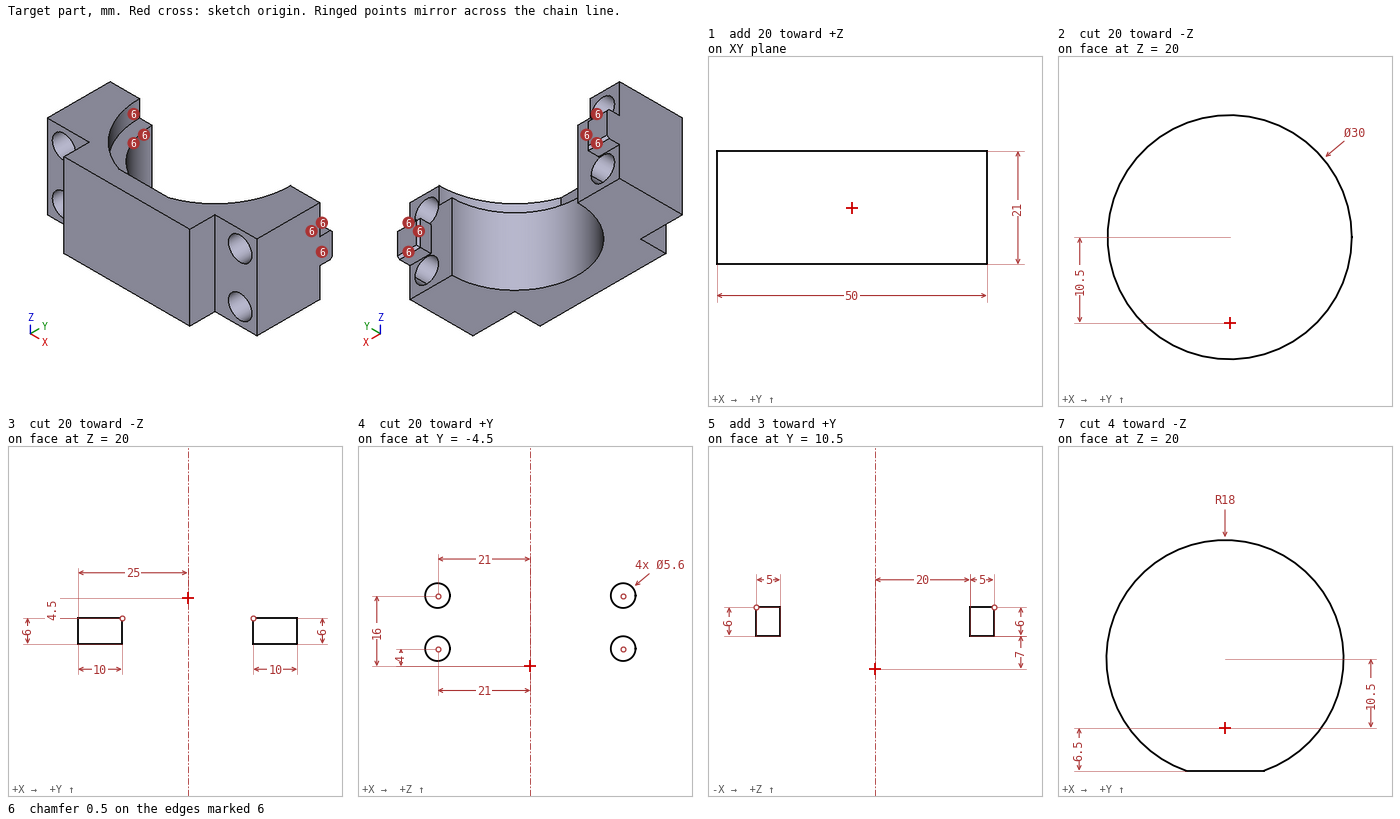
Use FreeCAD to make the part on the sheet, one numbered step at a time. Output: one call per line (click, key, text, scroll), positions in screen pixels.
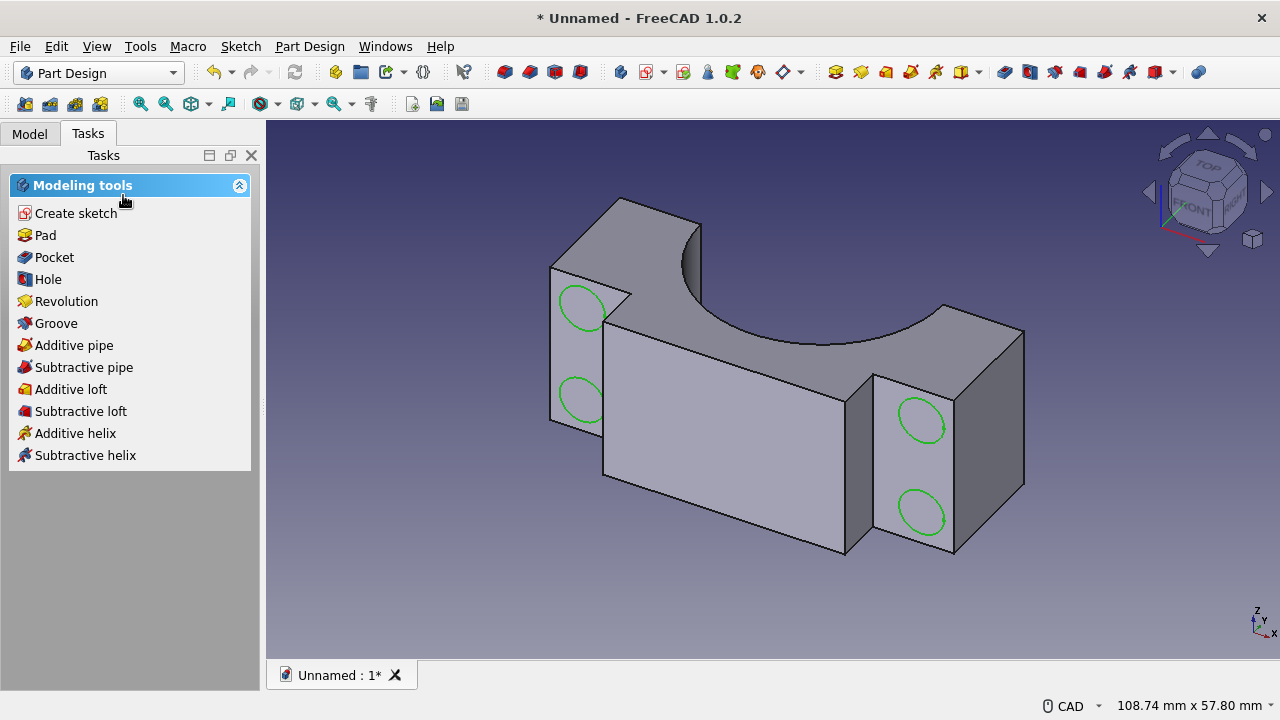
click(1005, 72)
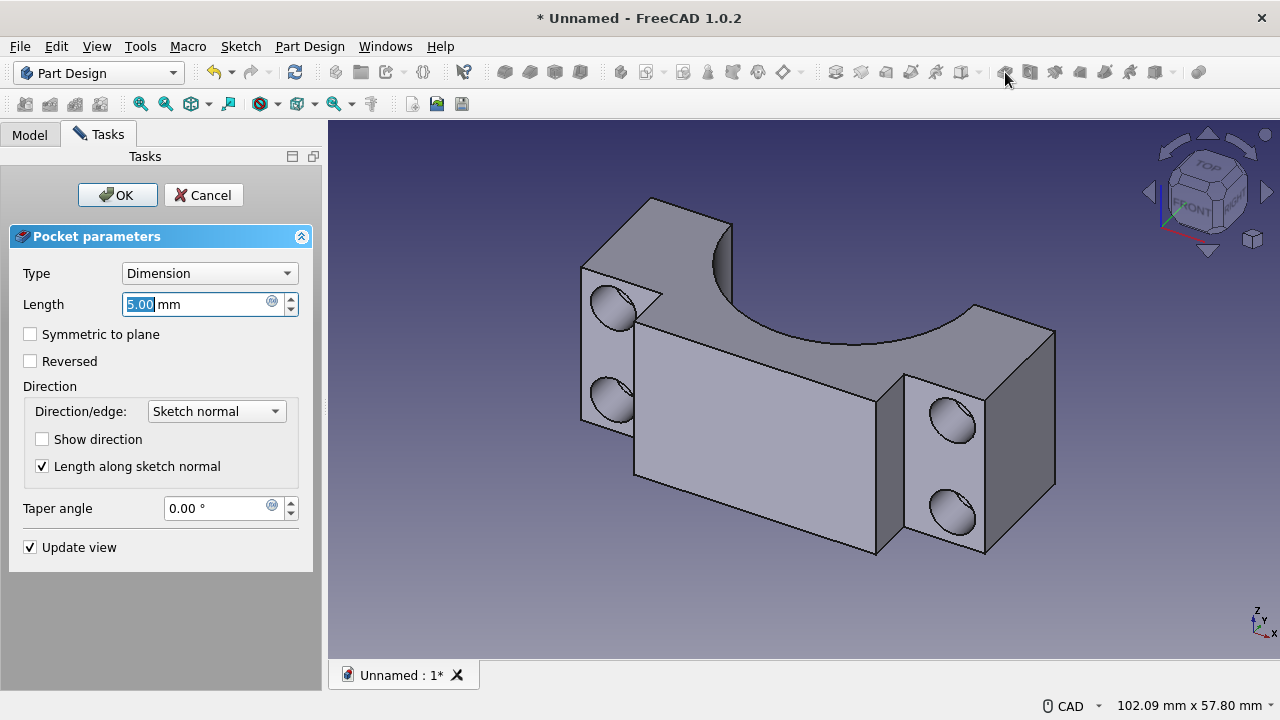
text(20)
key(Tab)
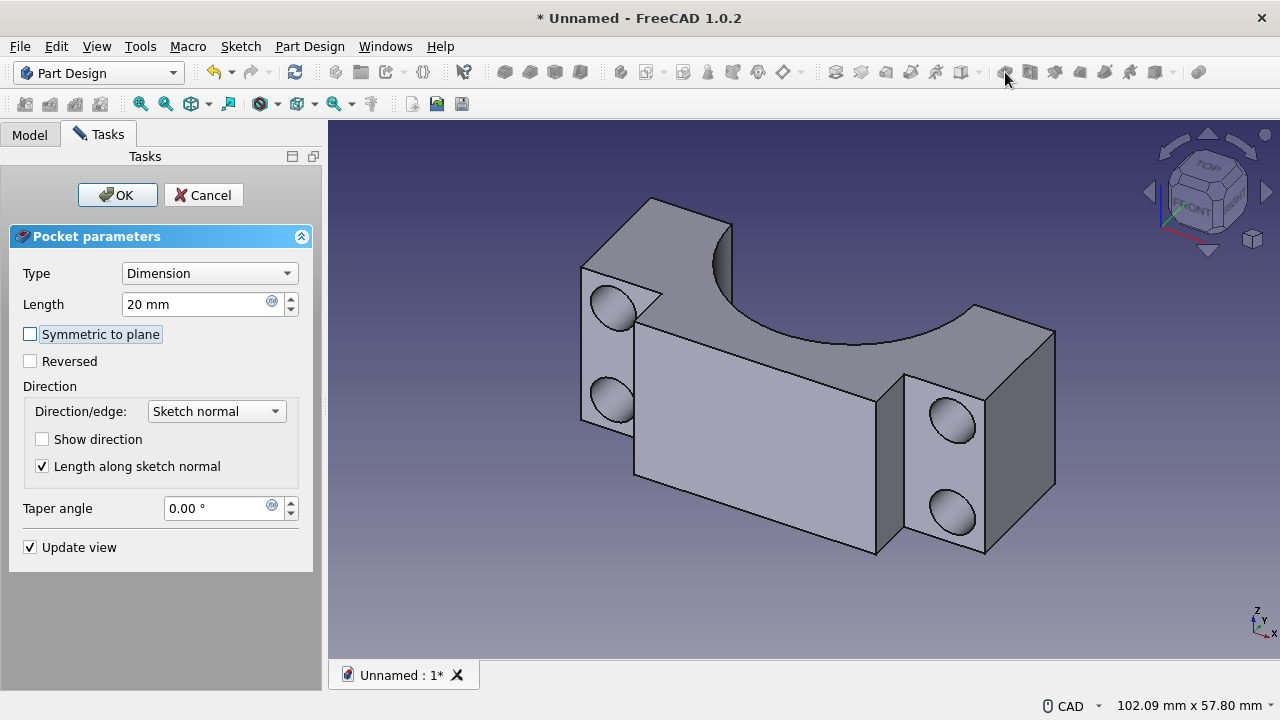
click(118, 195)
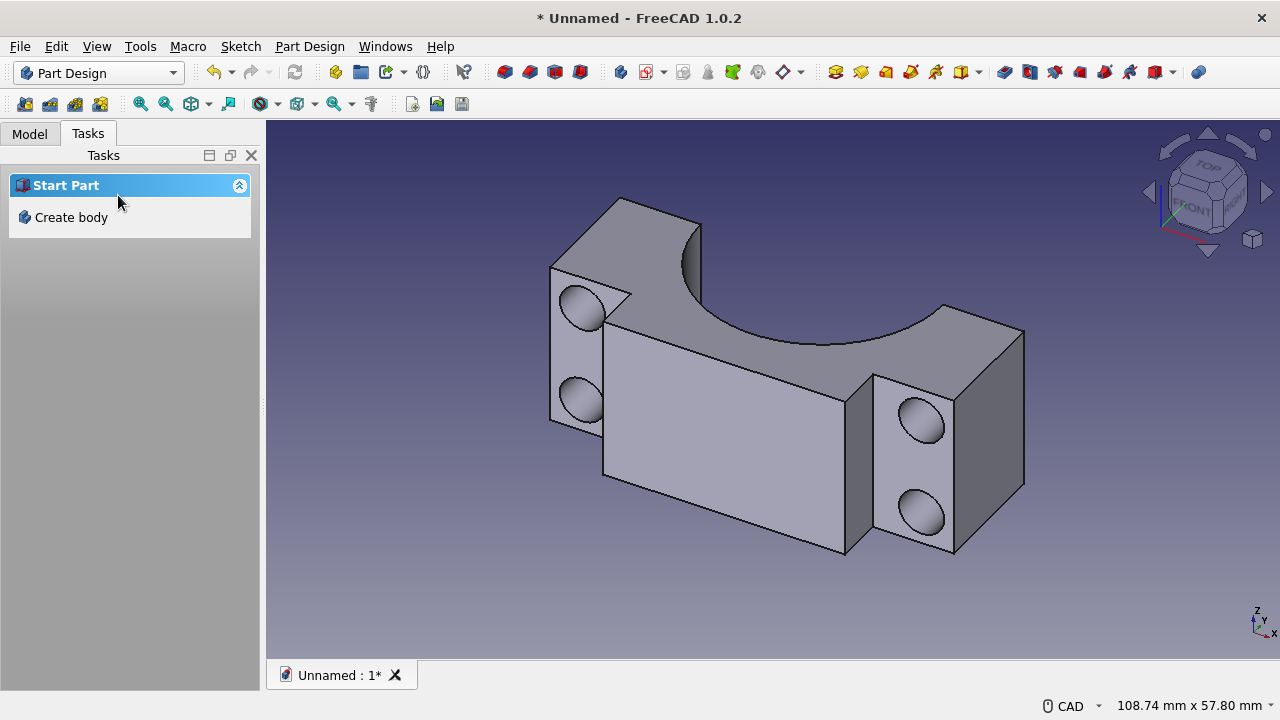
key(4)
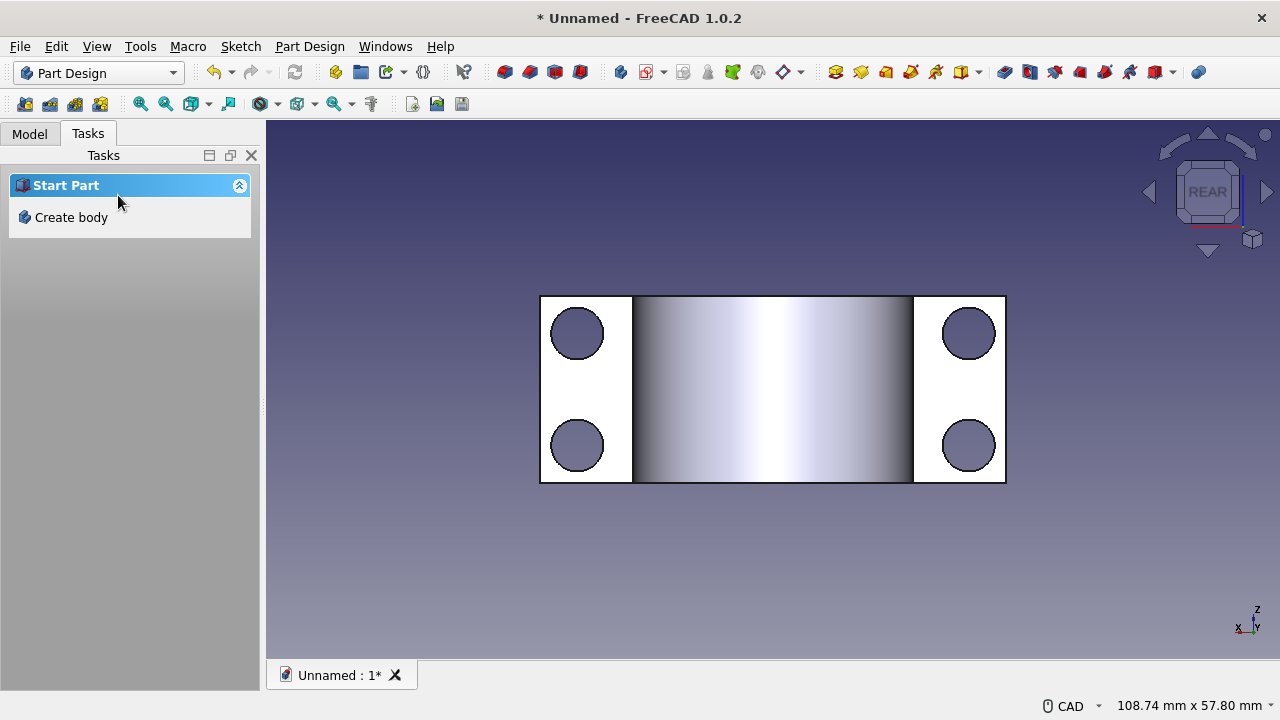
click(600, 389)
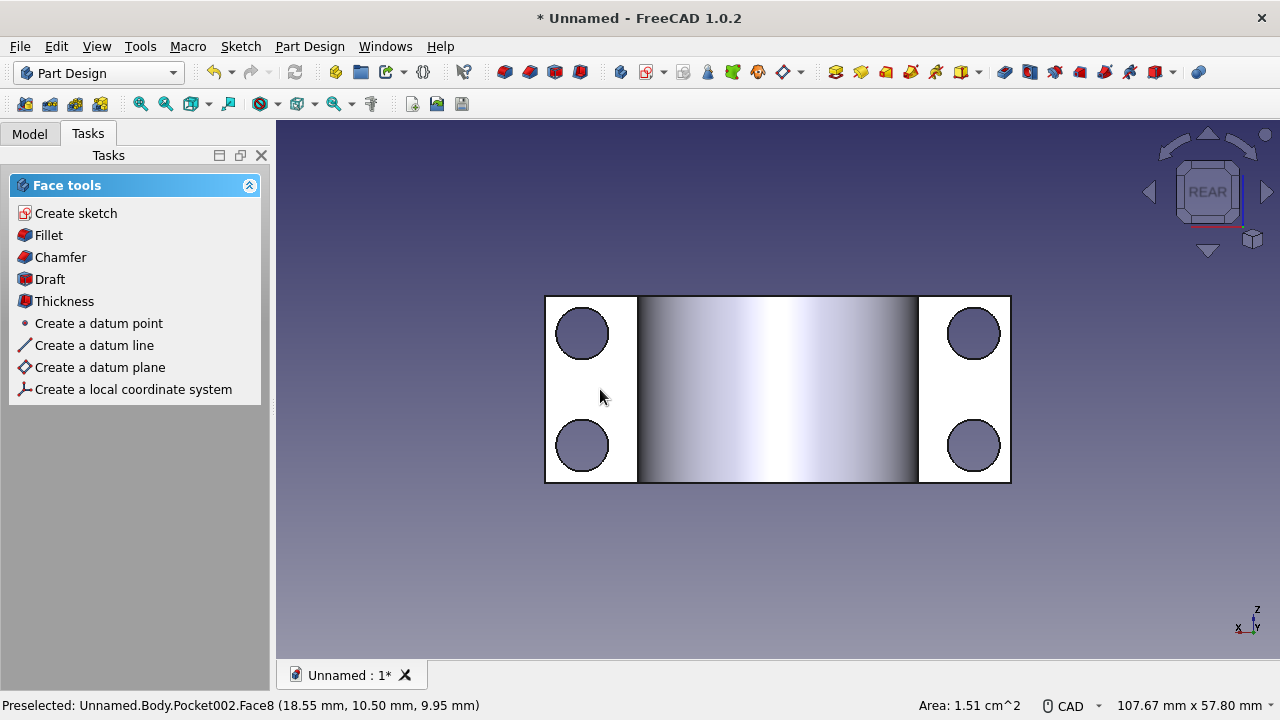
click(646, 72)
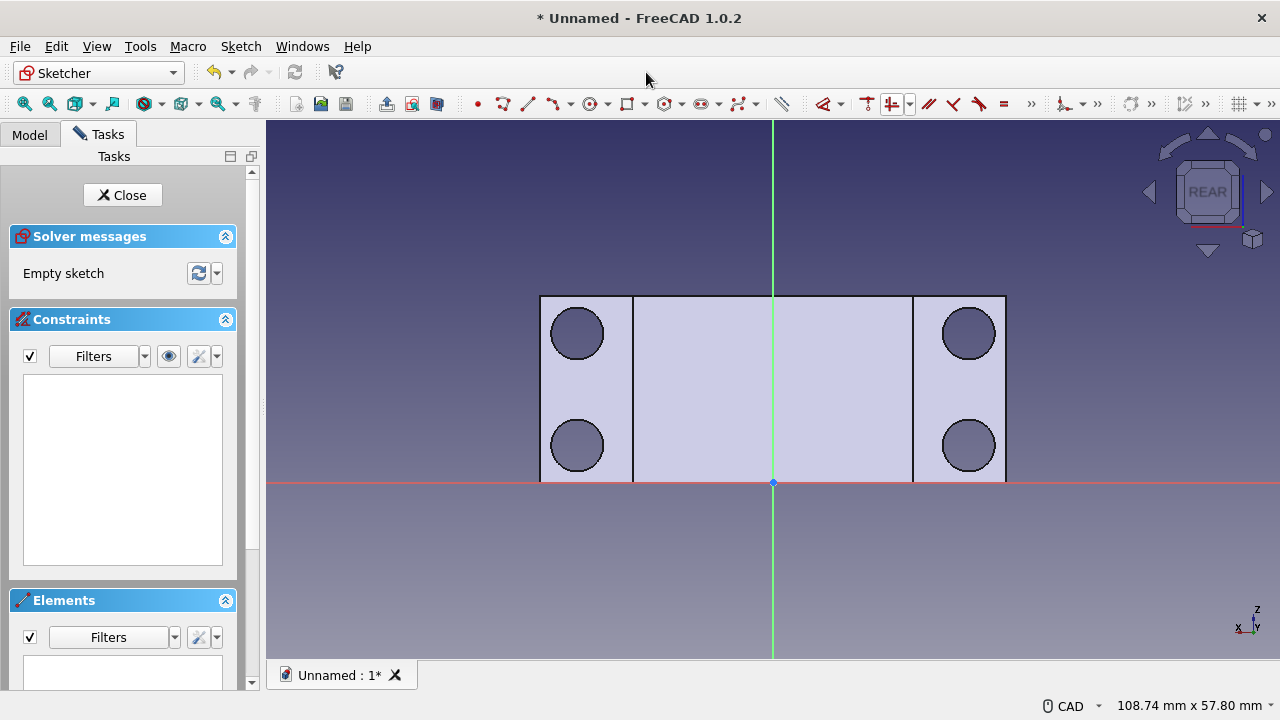
key(g)
key(r)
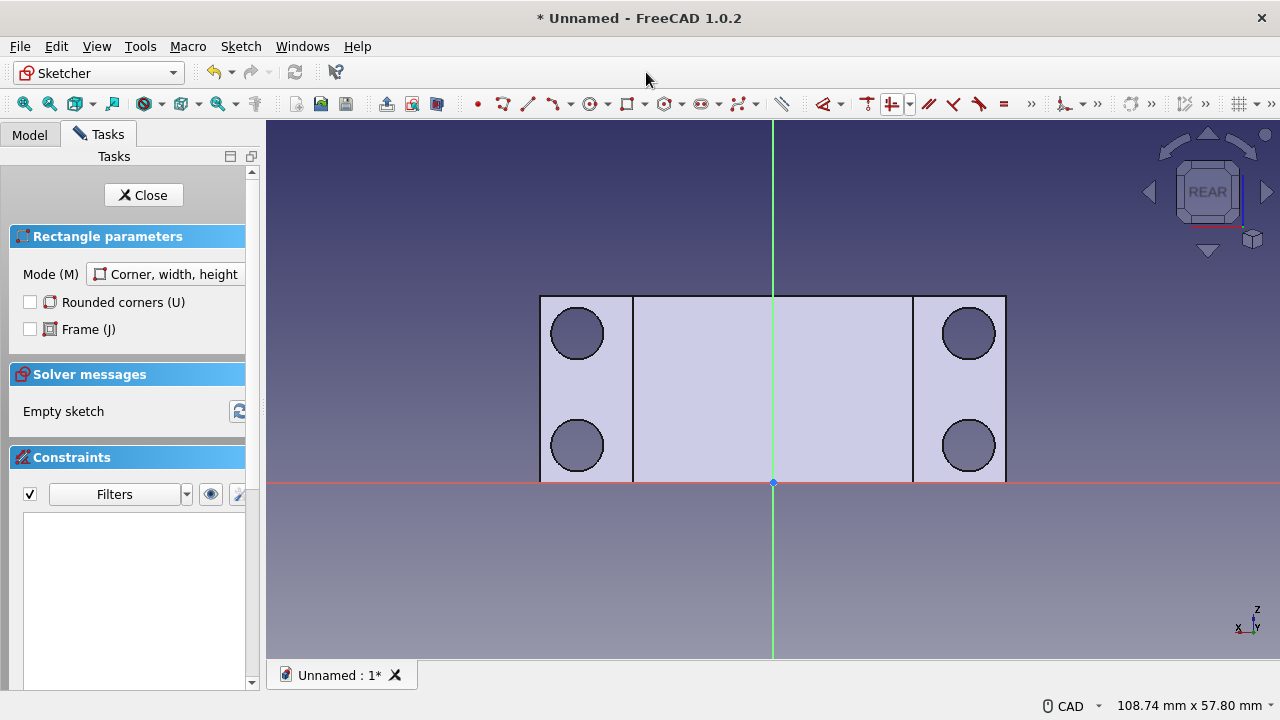
click(960, 362)
move(1006, 417)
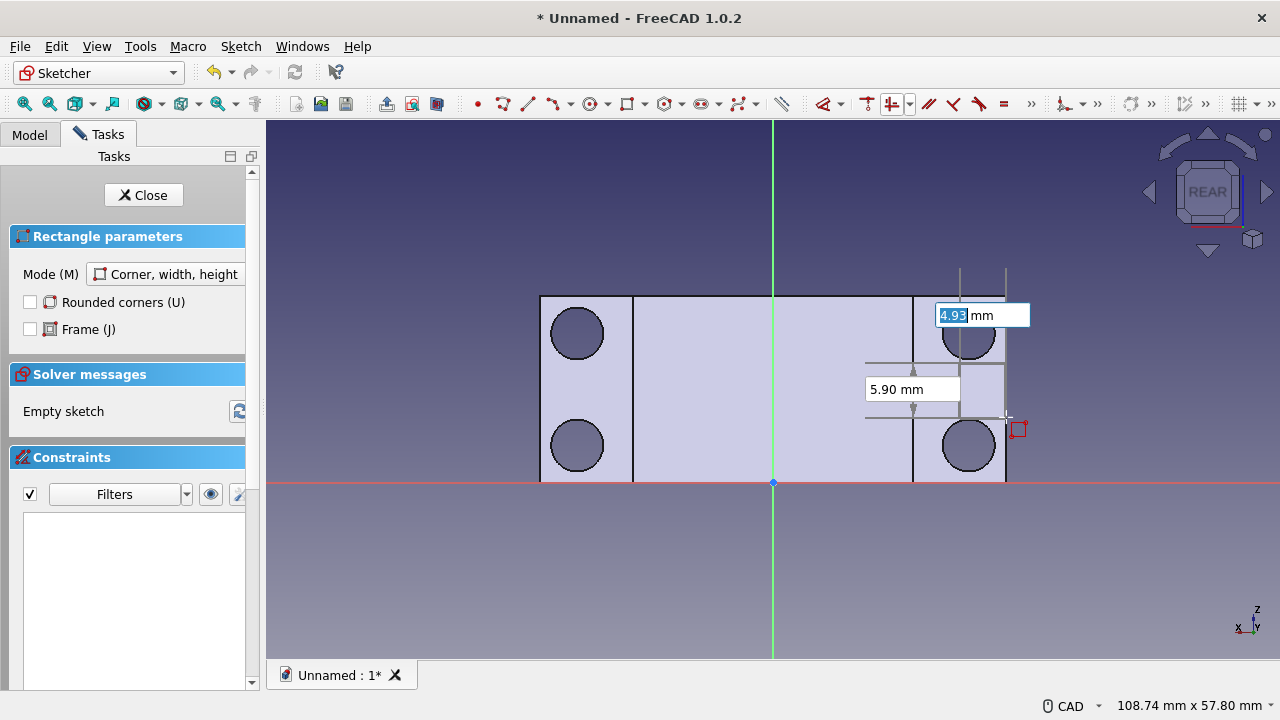
text(5)
key(Tab)
text(6)
key(Return)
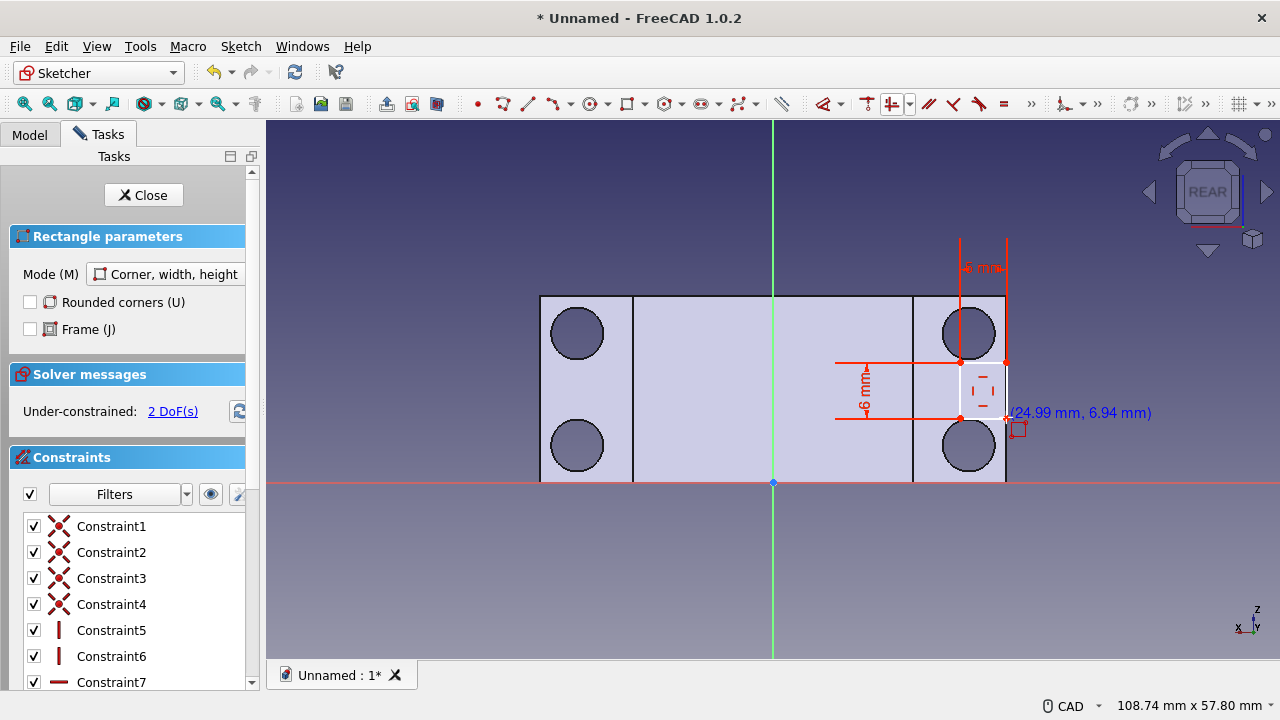
click(540, 362)
move(586, 417)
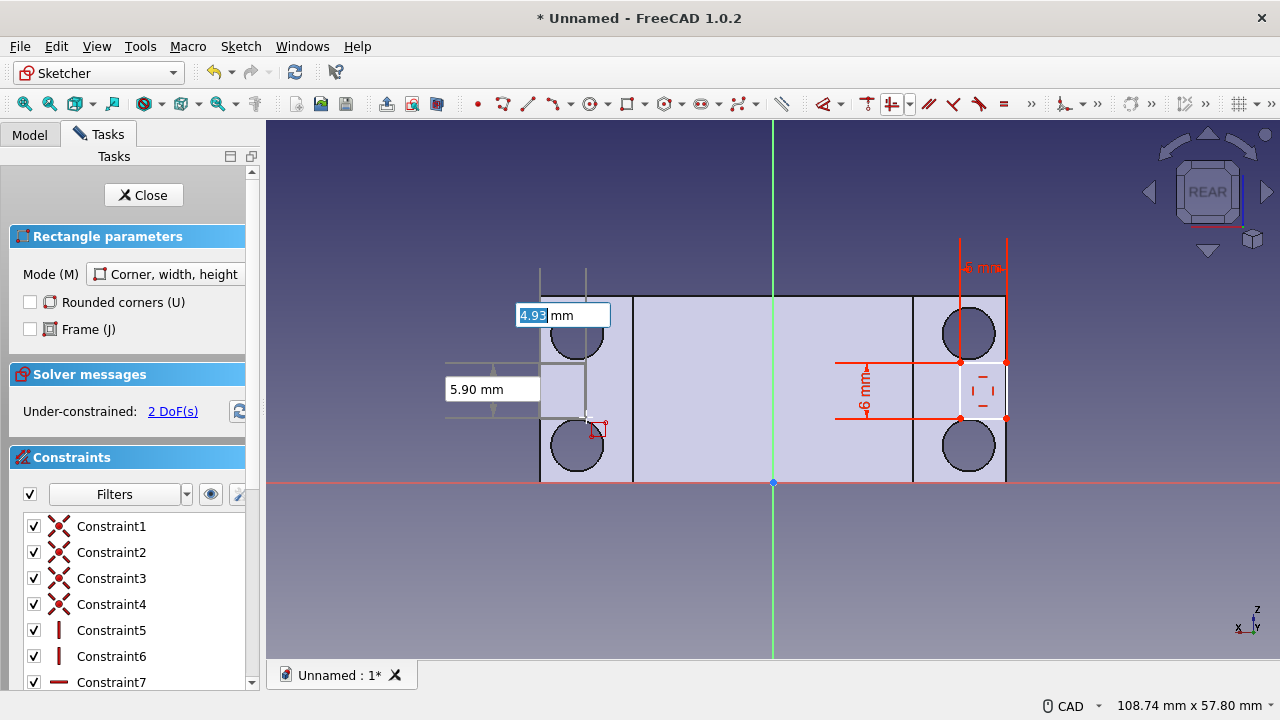
text(5)
key(Tab)
text(6)
key(Return)
key(Escape)